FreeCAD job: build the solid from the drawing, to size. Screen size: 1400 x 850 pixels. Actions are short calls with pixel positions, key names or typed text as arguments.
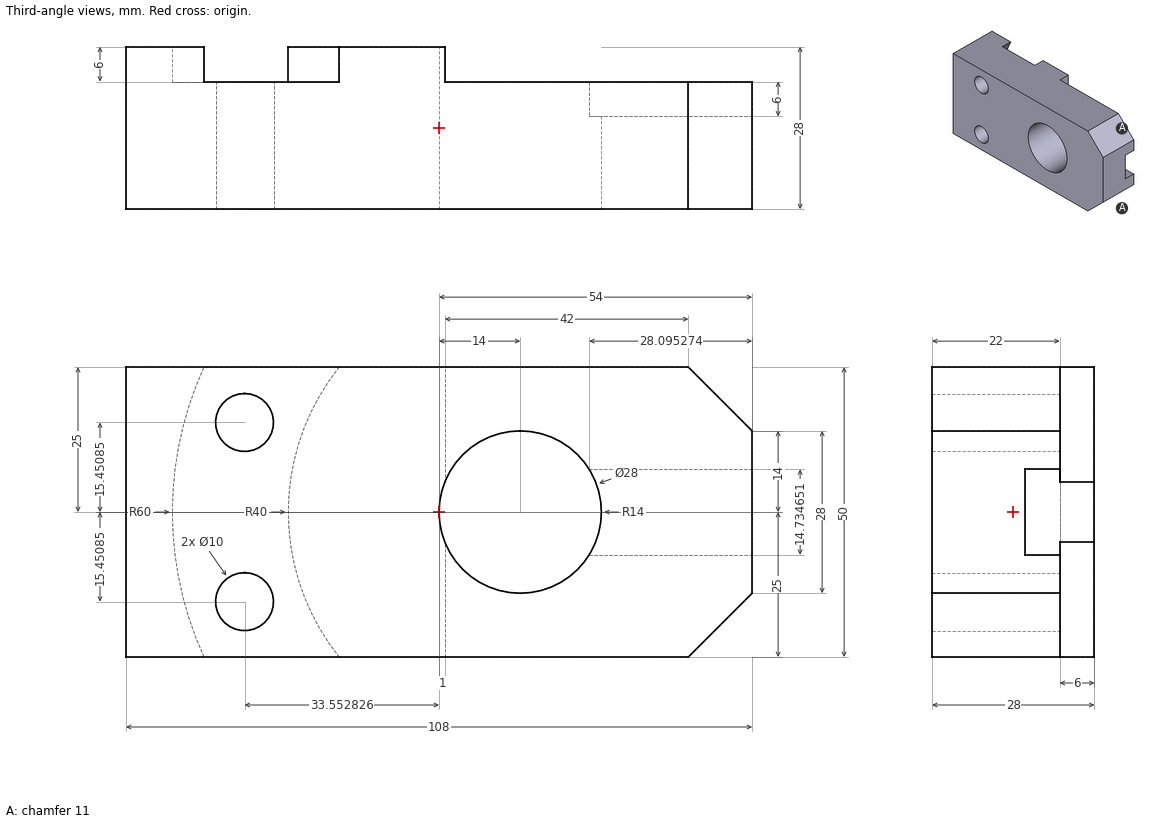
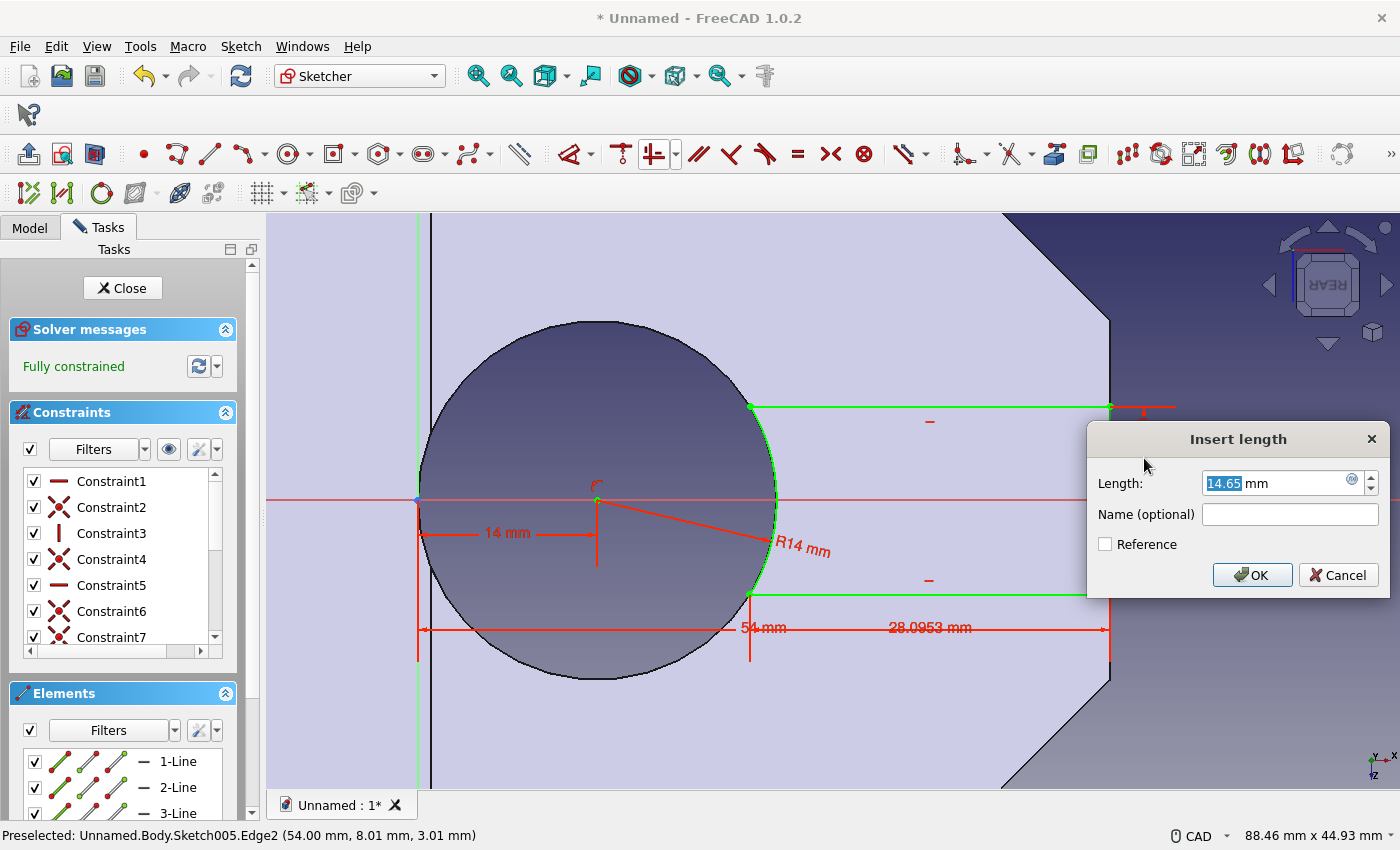
text(14.734651)
key(Return)
key(Escape)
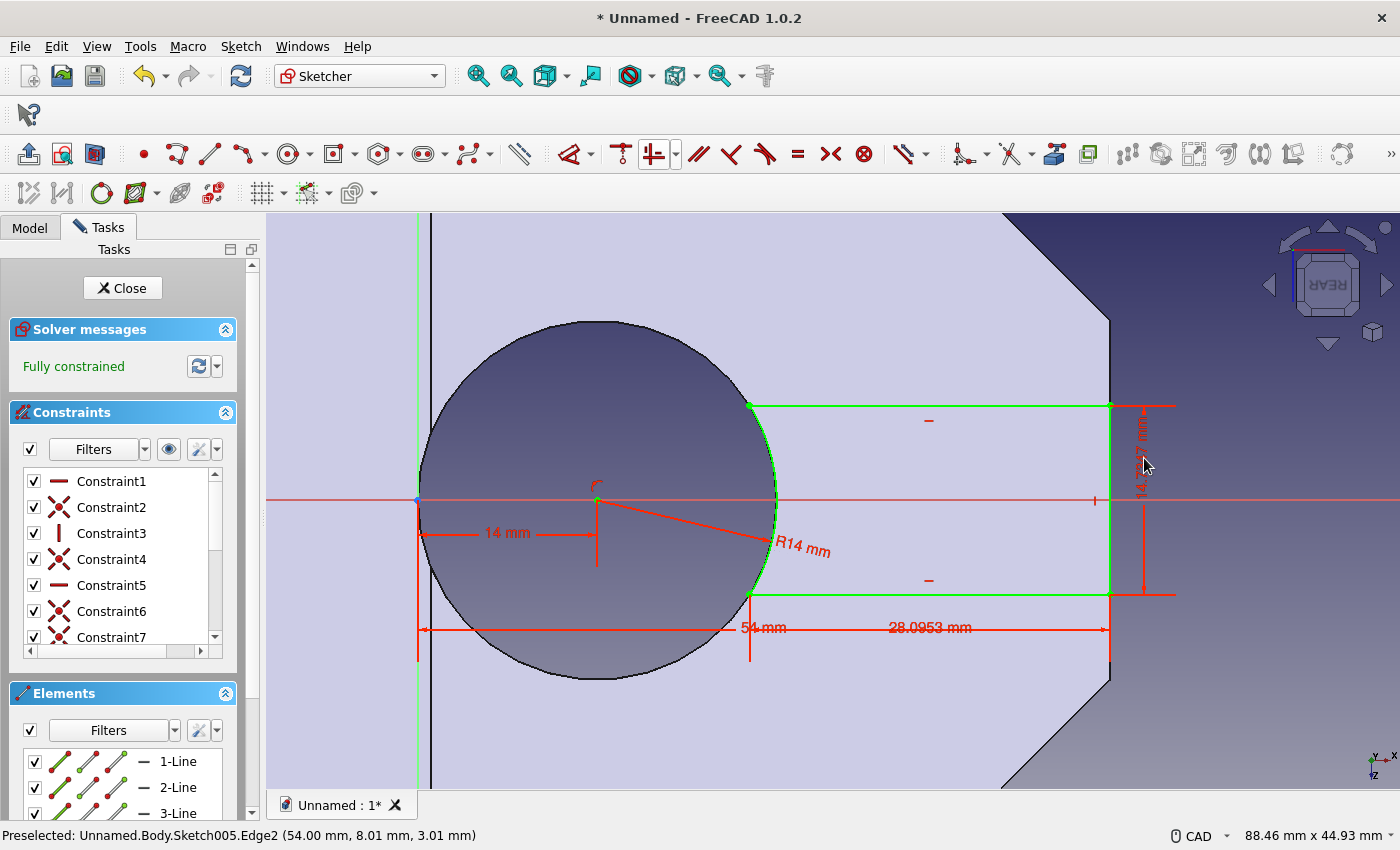
click(123, 288)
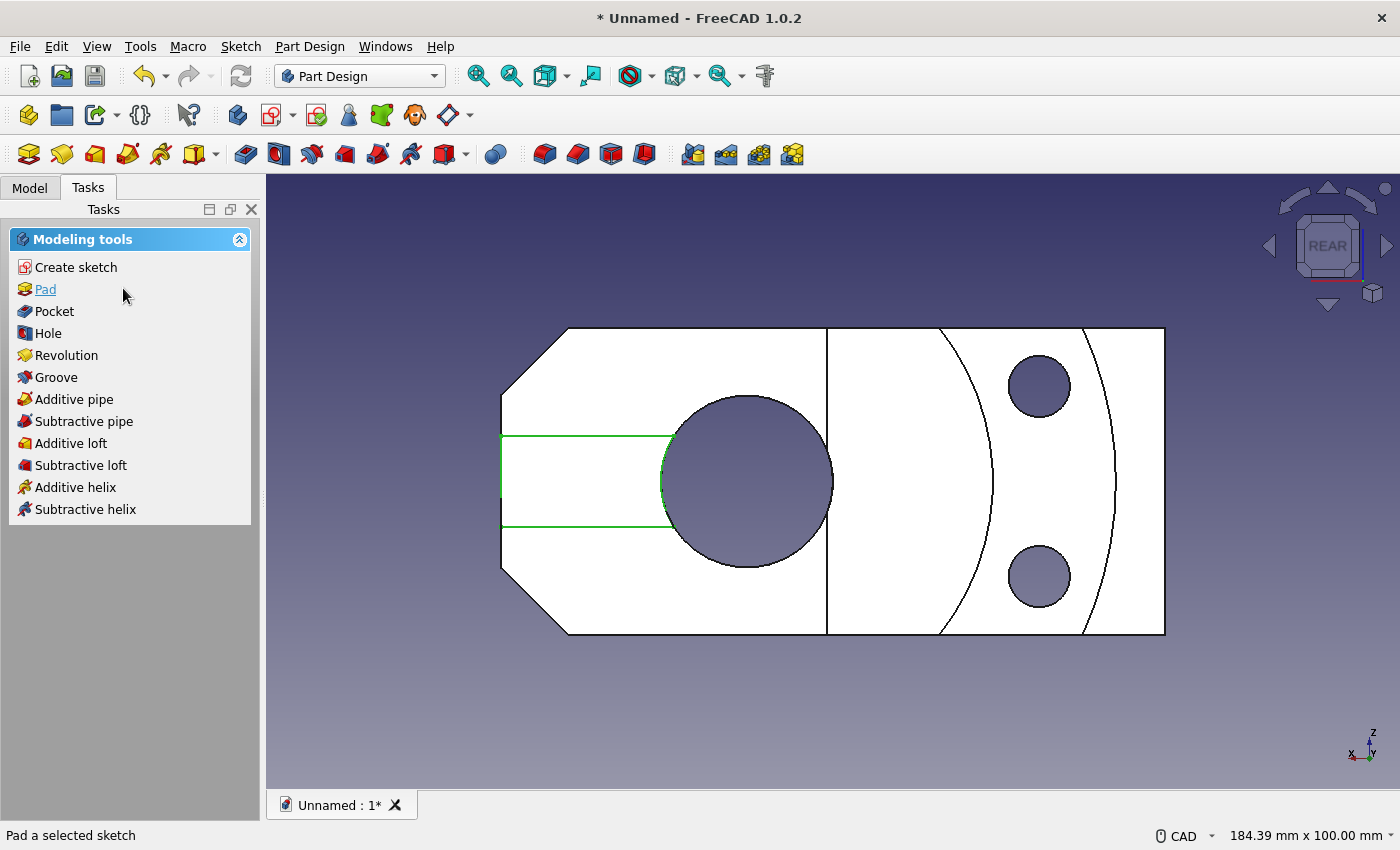
click(246, 154)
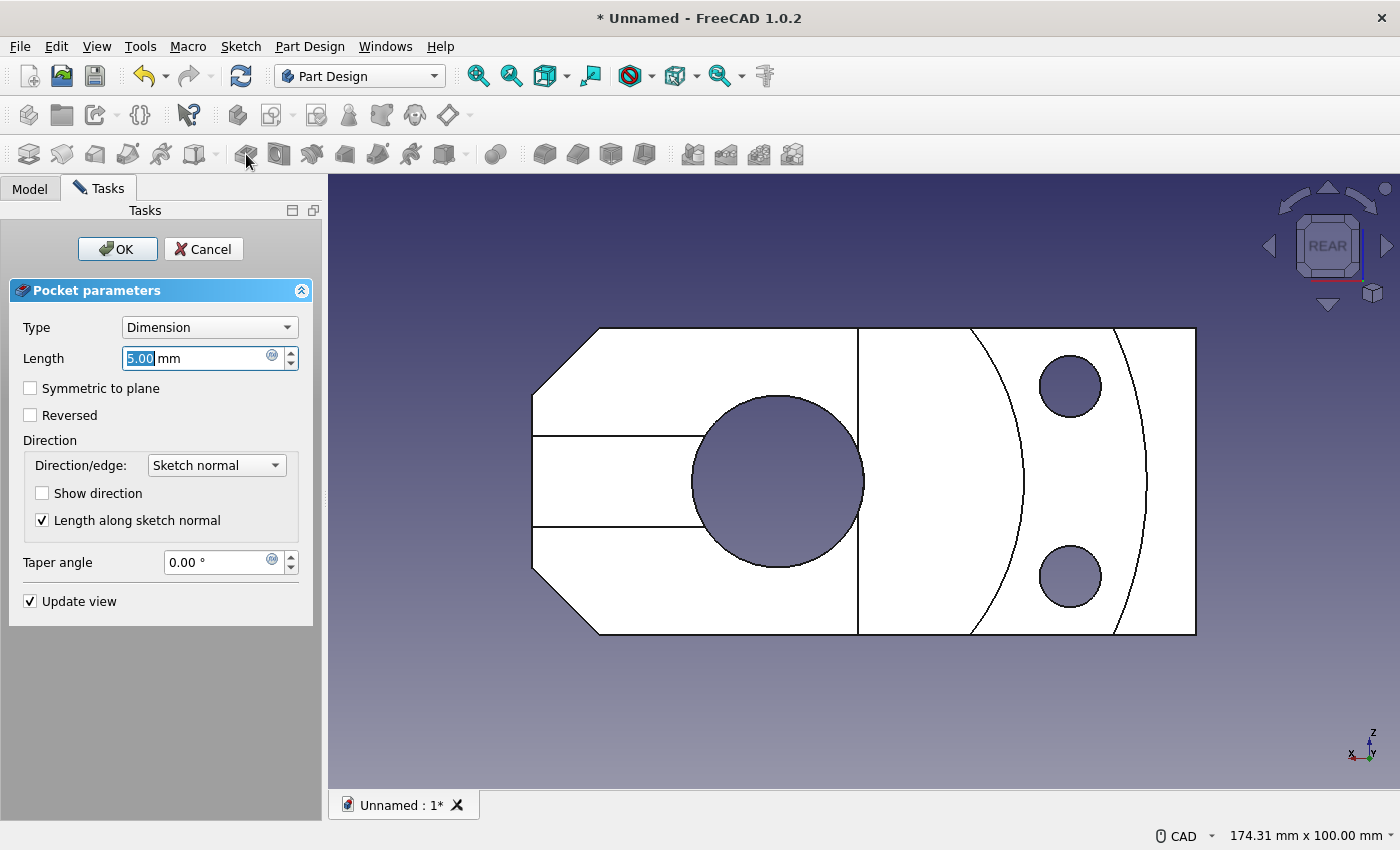
text(6)
key(Tab)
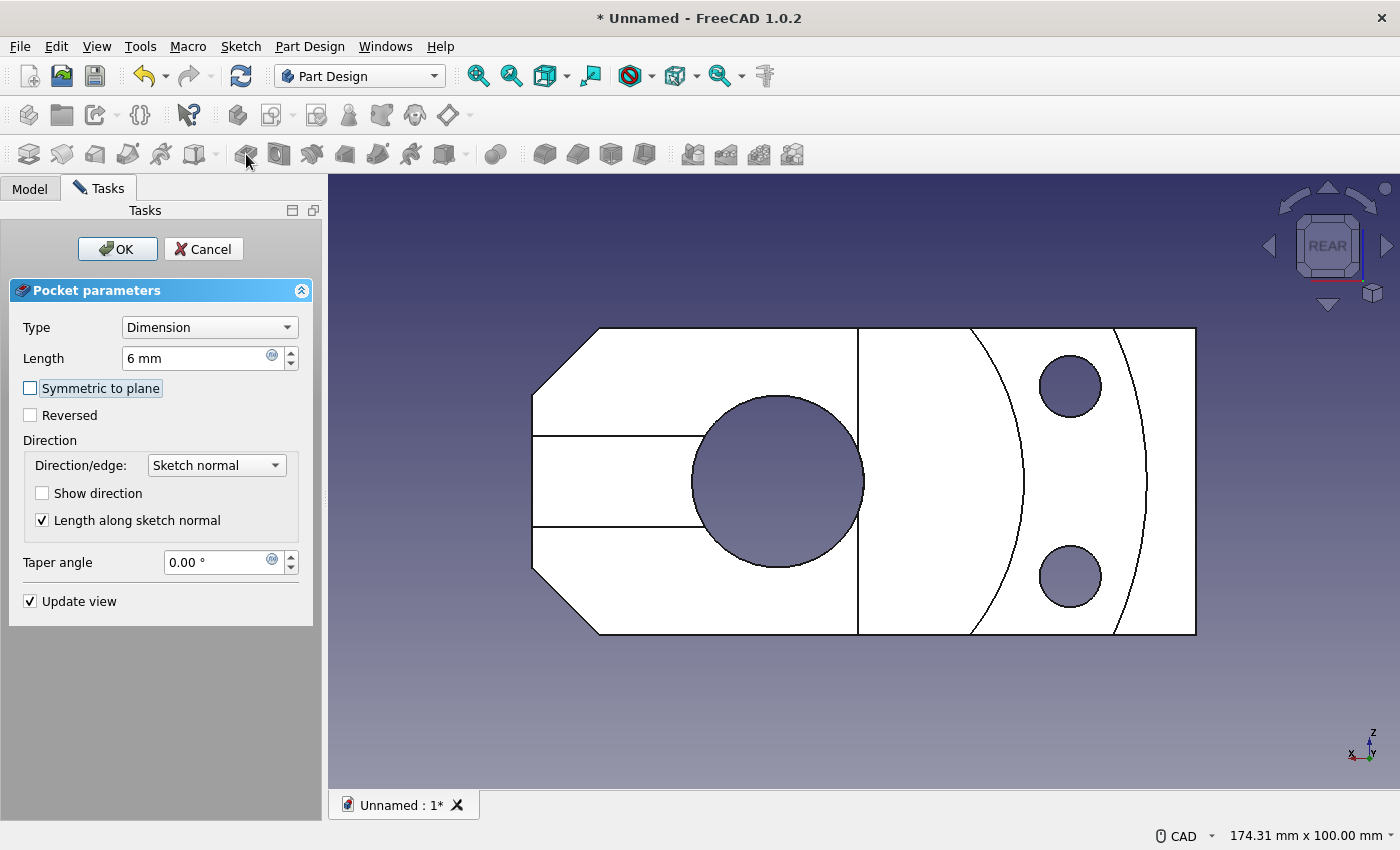
click(118, 249)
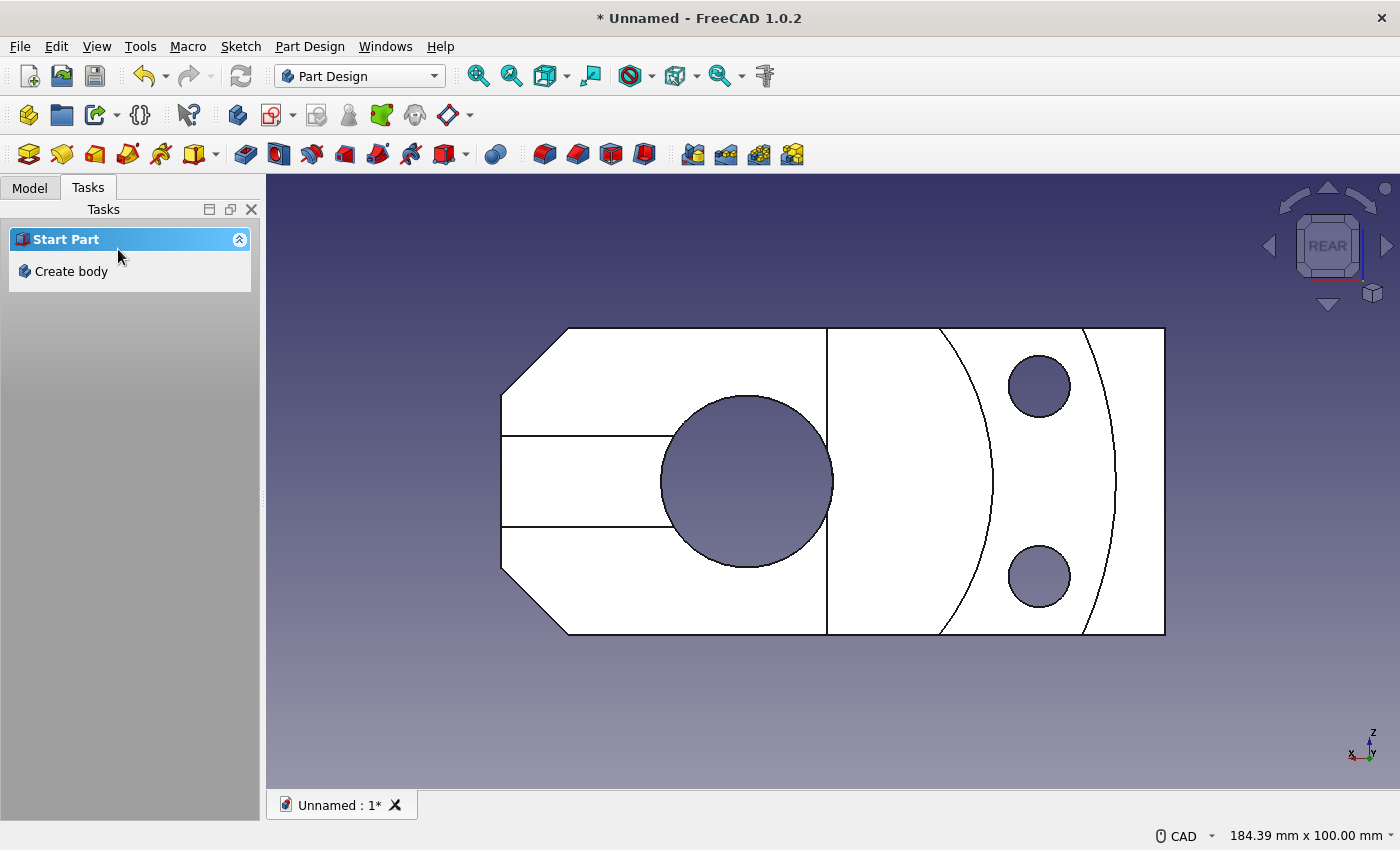
key(0)